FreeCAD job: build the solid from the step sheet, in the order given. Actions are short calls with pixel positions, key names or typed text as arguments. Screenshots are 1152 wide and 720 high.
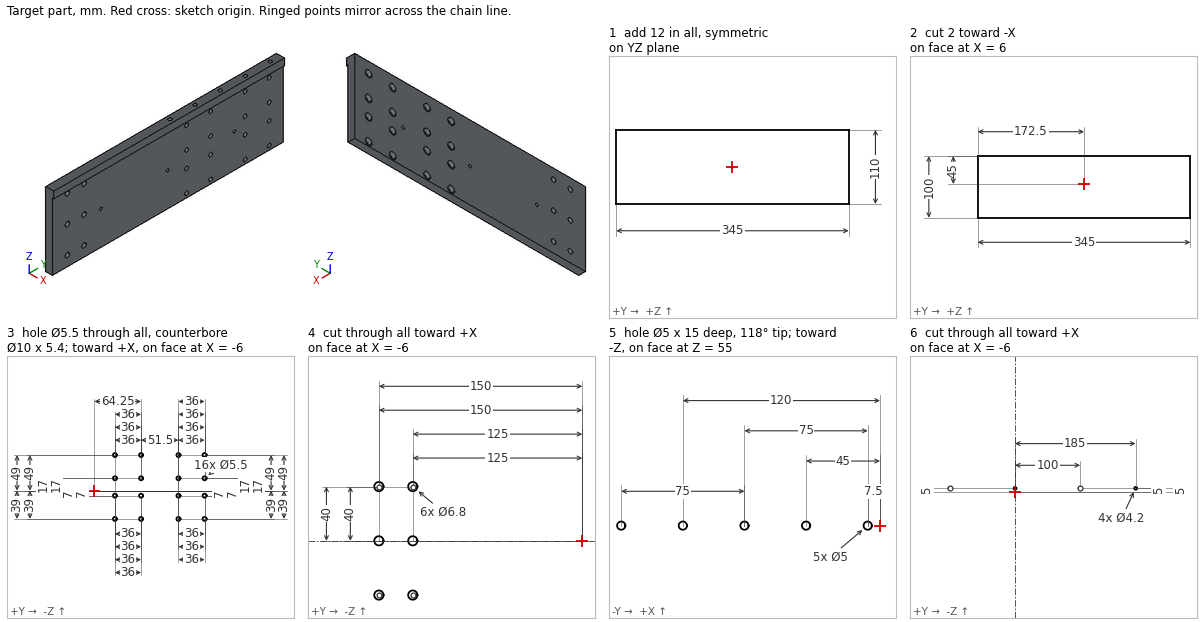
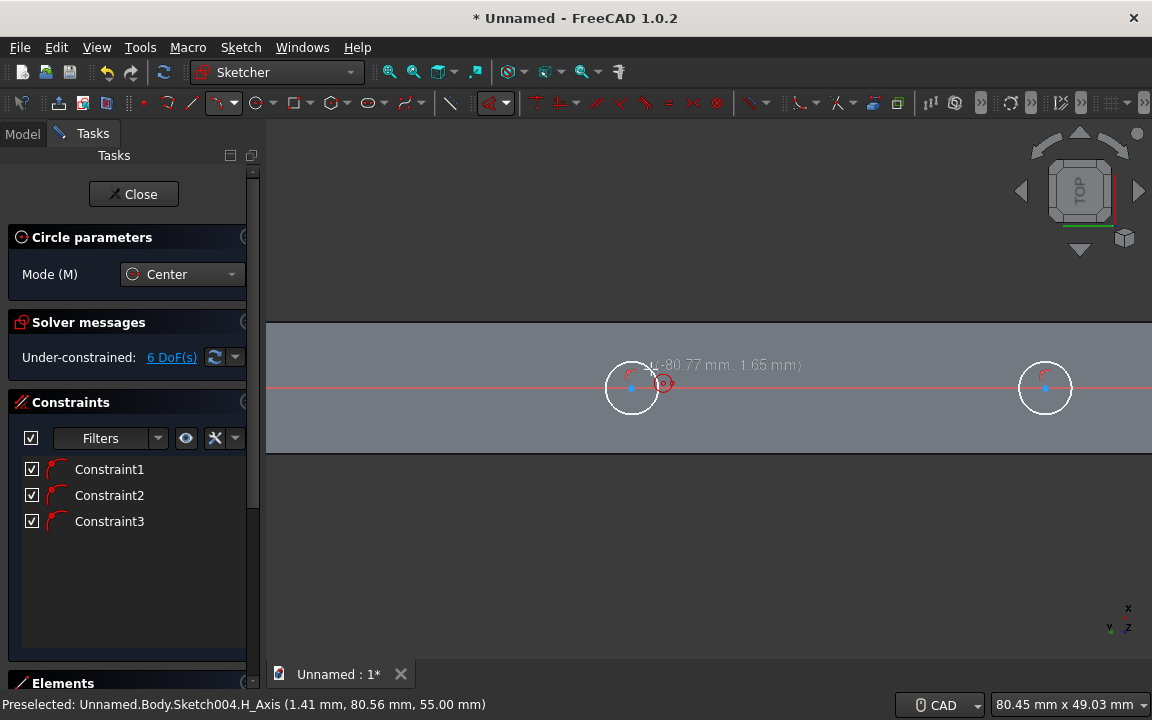
scroll(632, 389, down, 6)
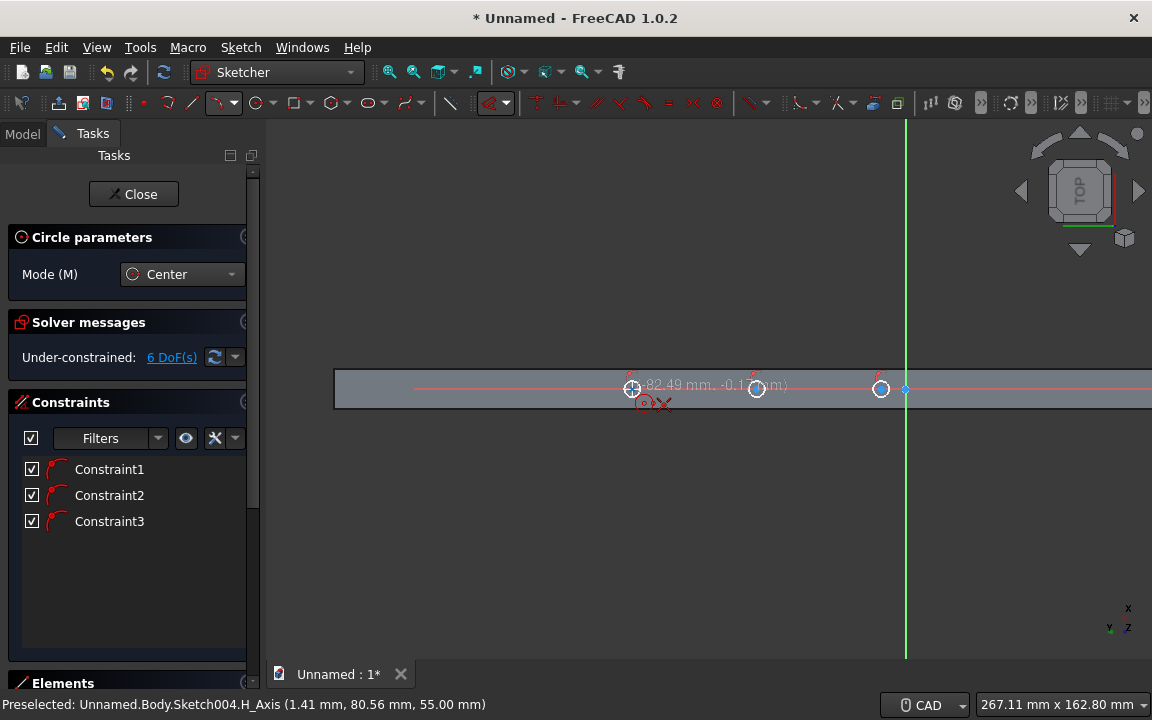
scroll(508, 389, up, 6)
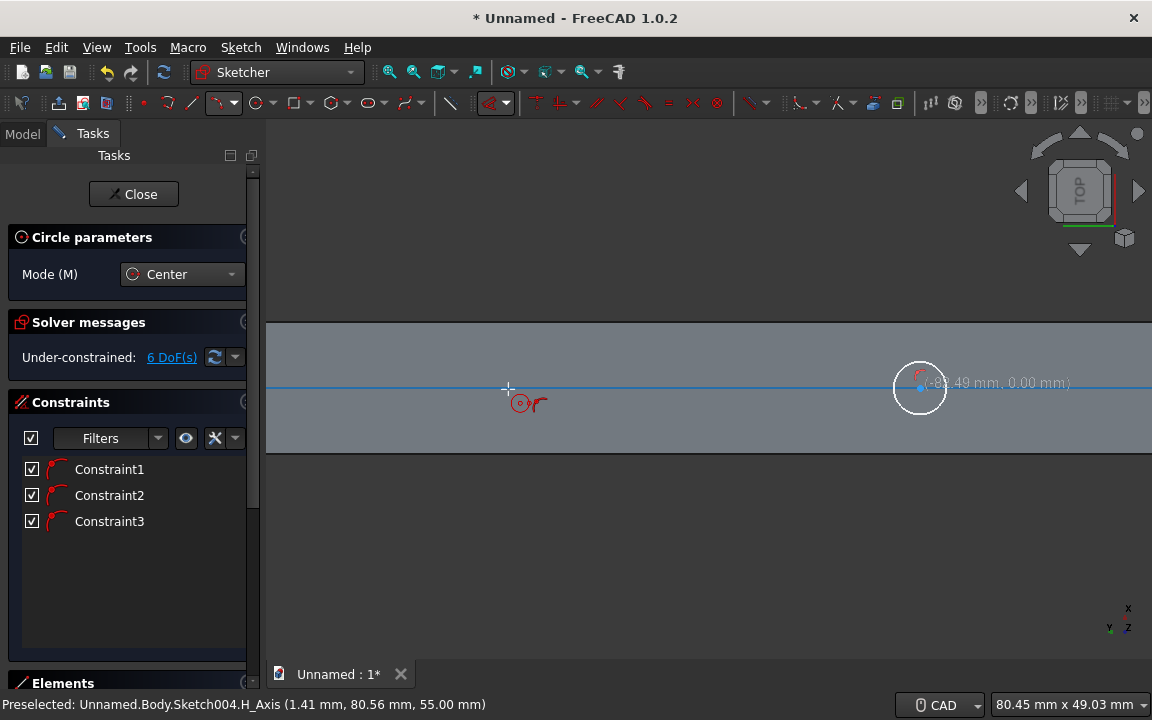
click(507, 388)
click(526, 369)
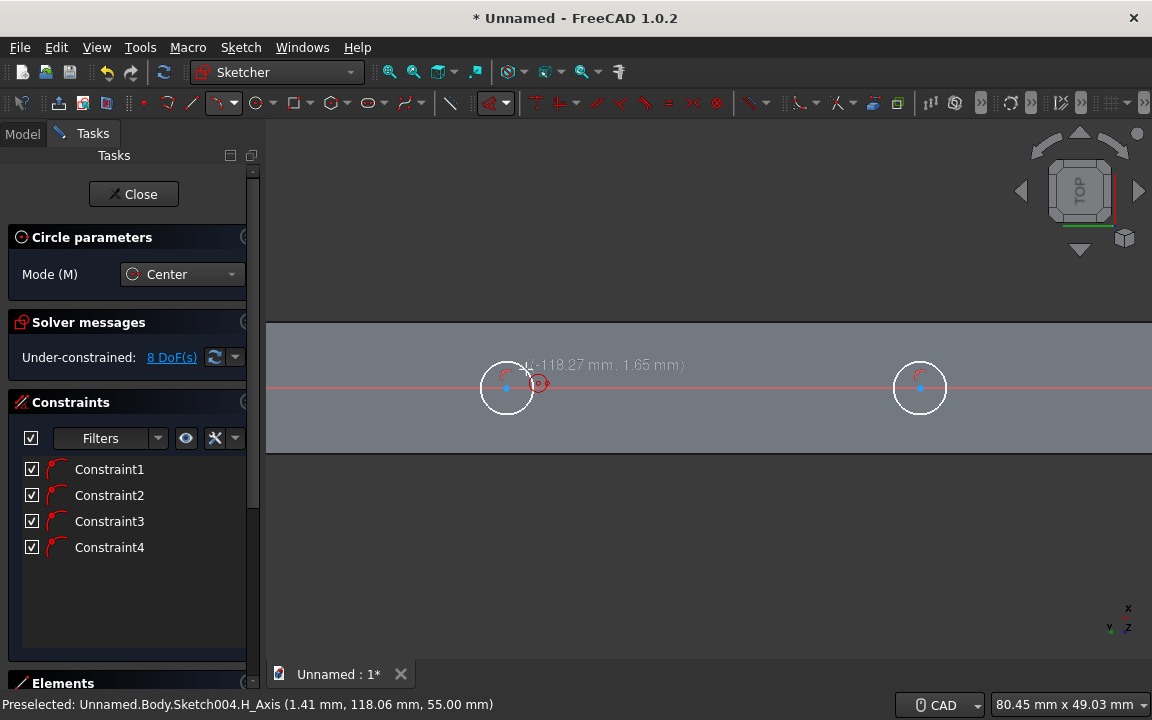
scroll(508, 389, down, 6)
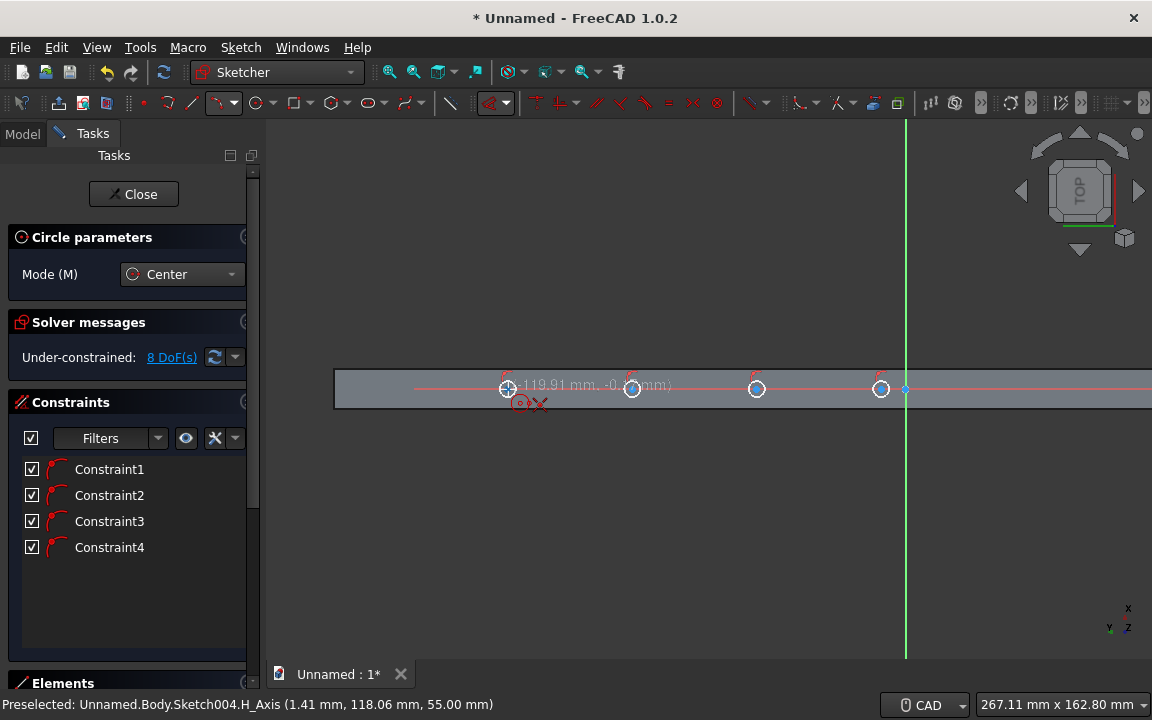
scroll(383, 389, up, 6)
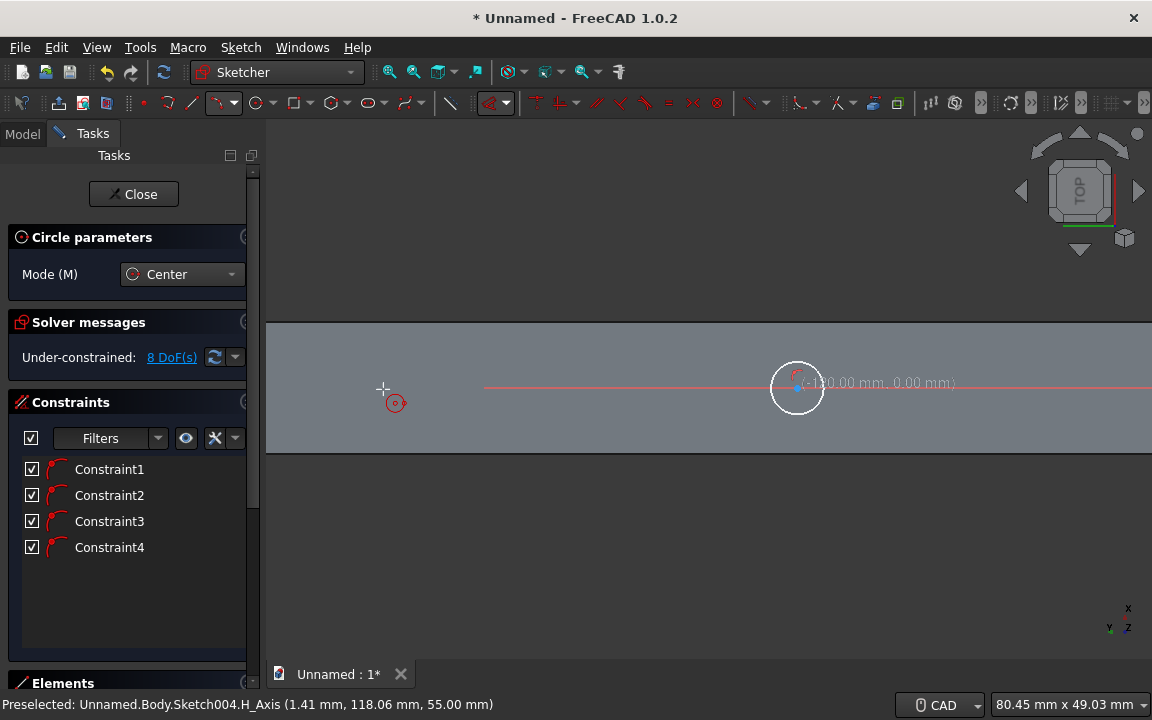
click(384, 388)
click(404, 369)
key(Escape)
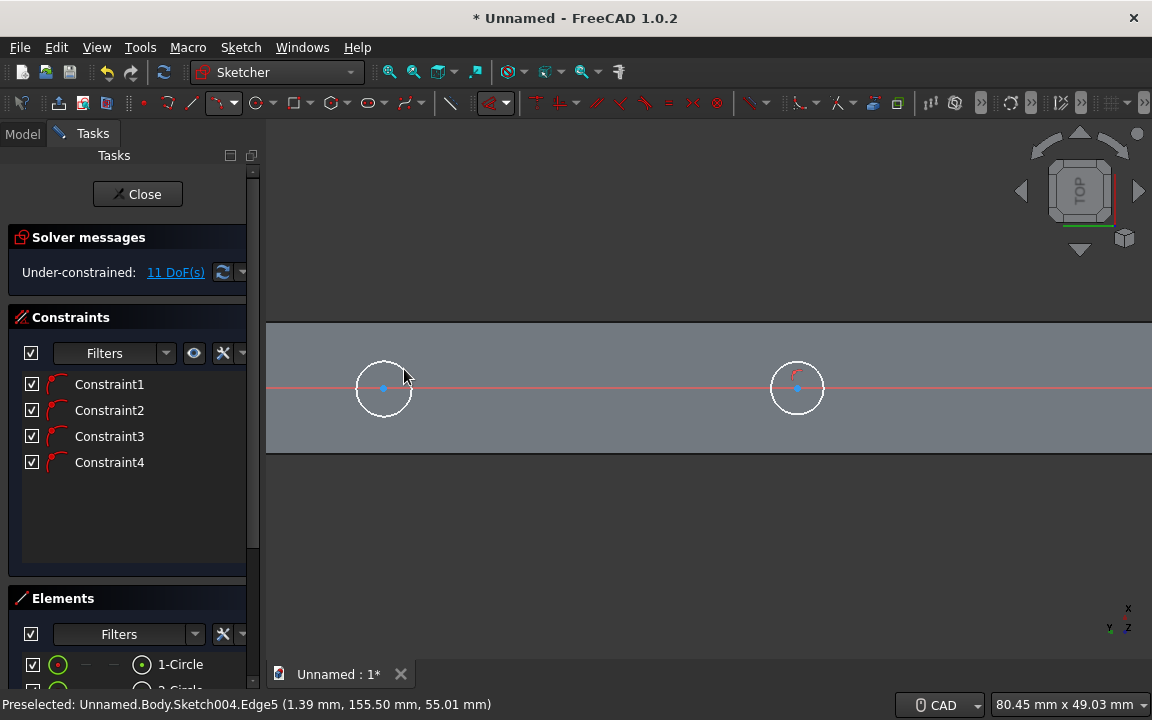
scroll(383, 389, down, 6)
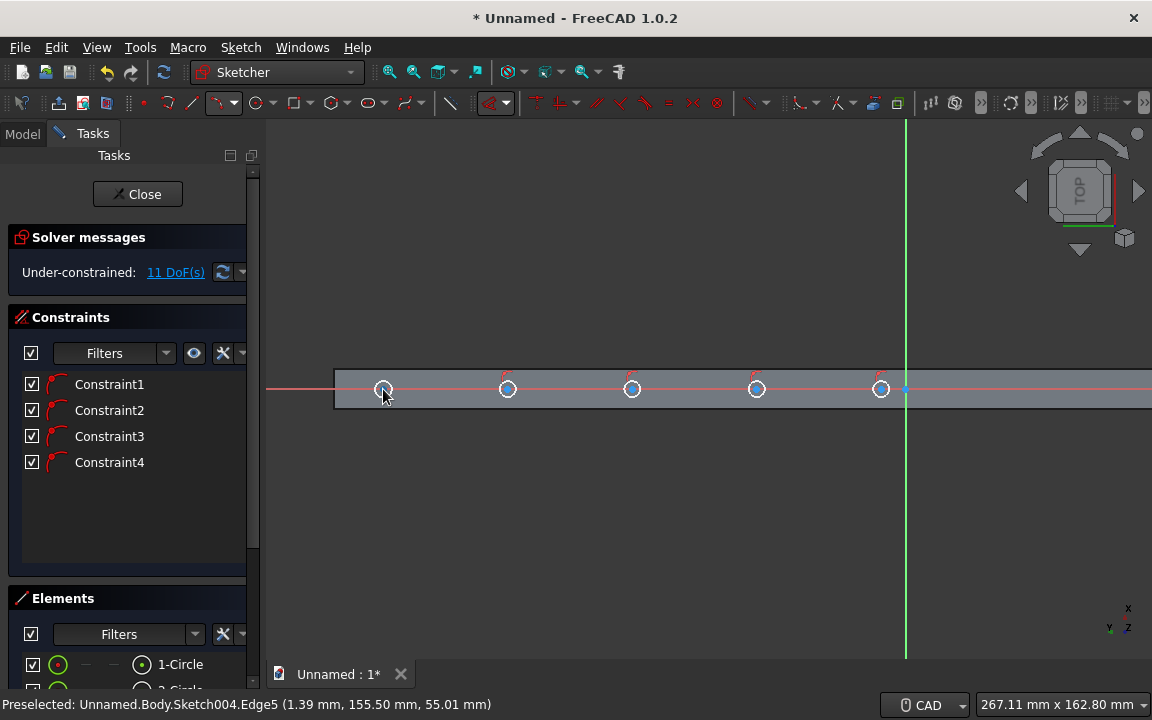
scroll(887, 383, up, 5)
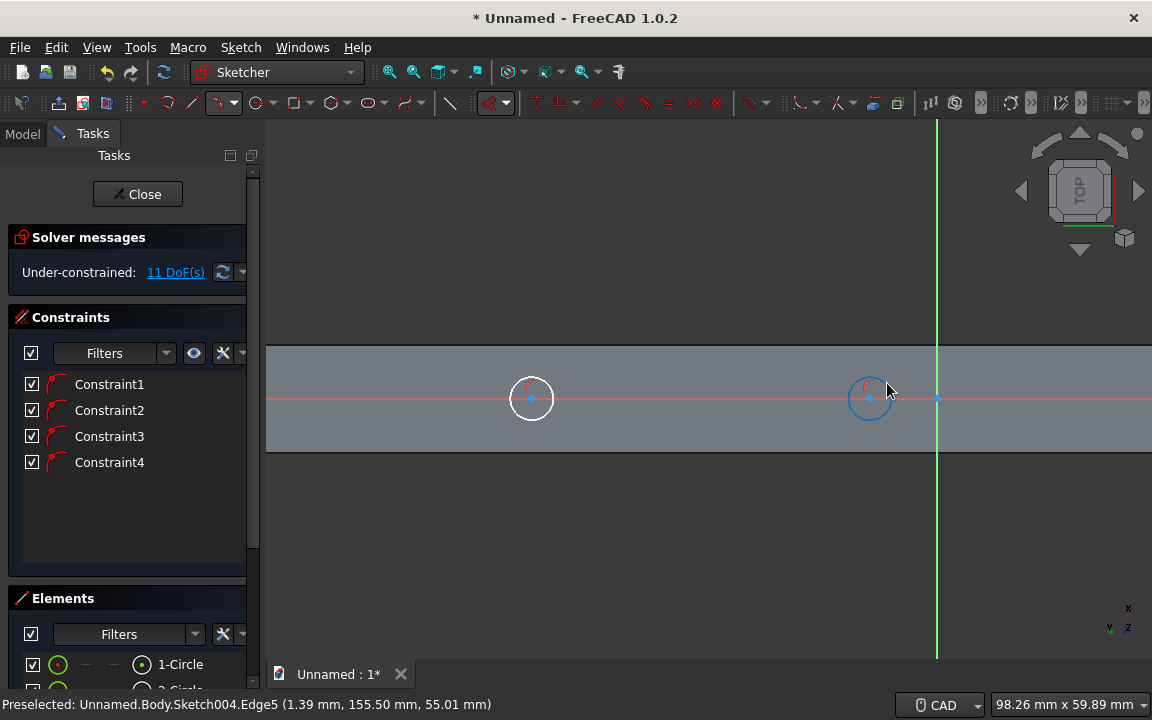
click(885, 383)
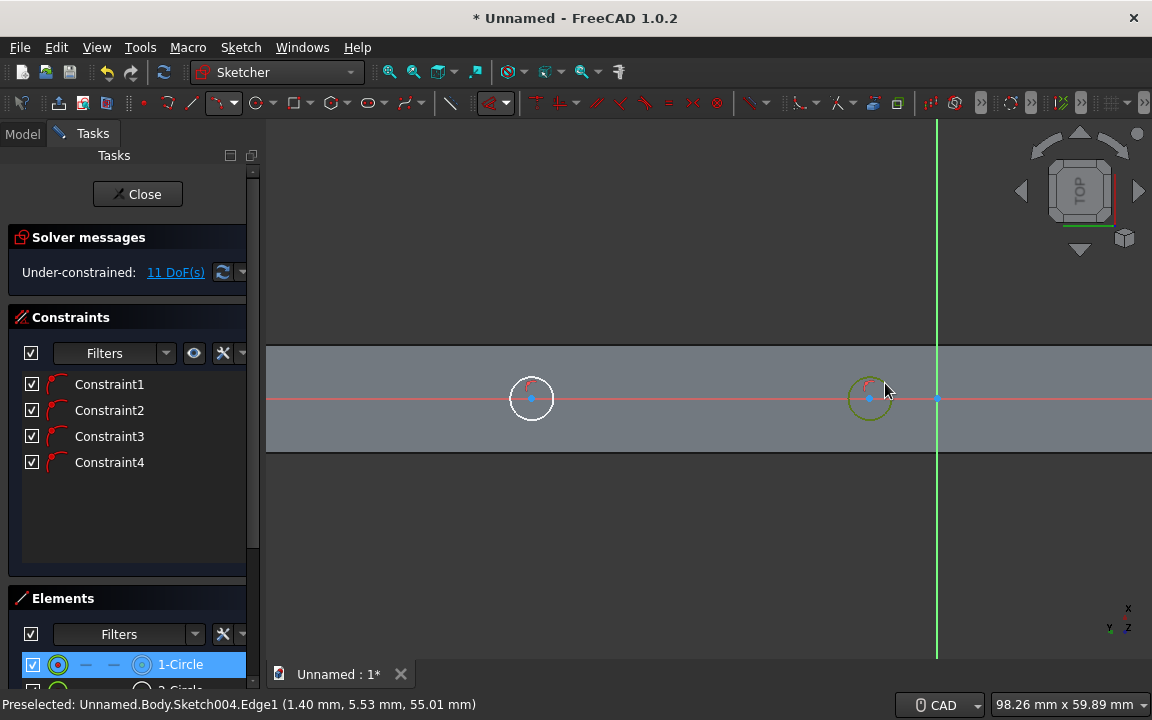
click(547, 383)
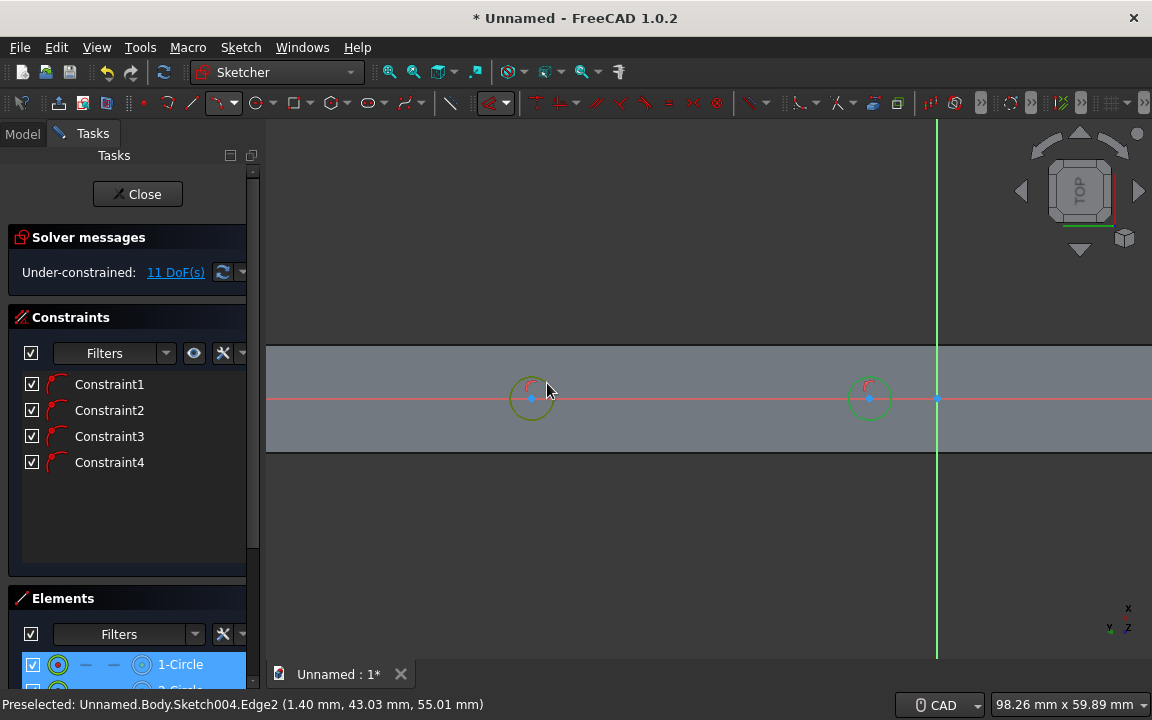
scroll(888, 383, down, 5)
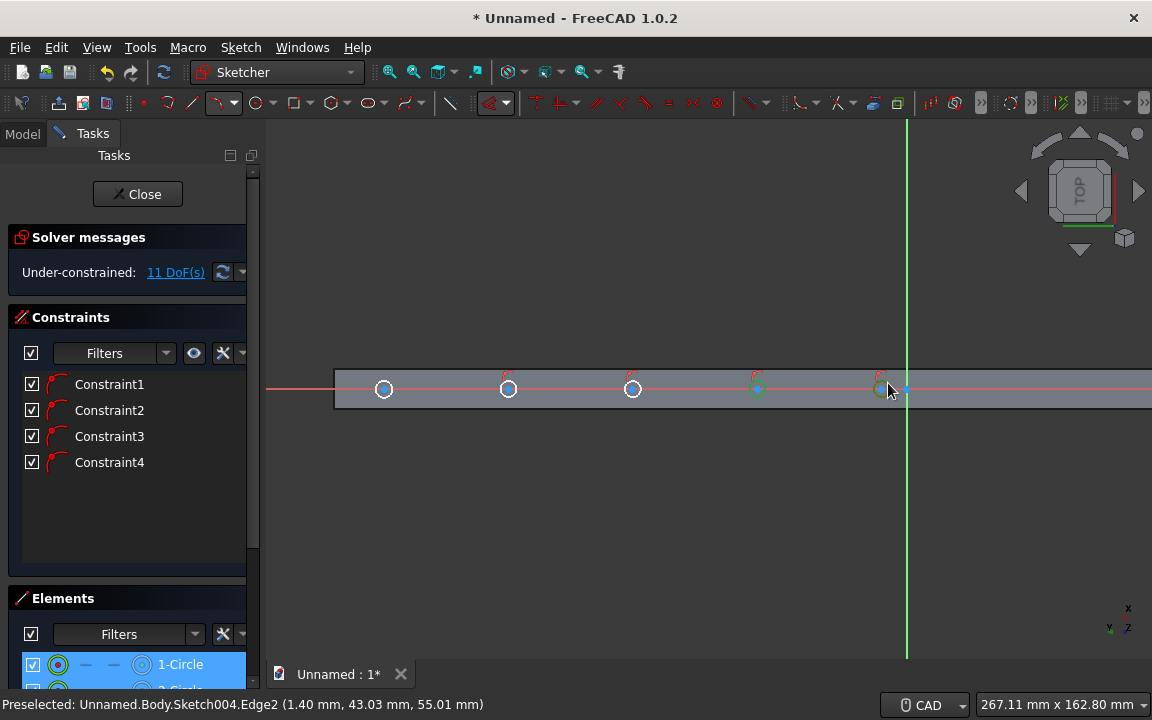
scroll(638, 383, up, 5)